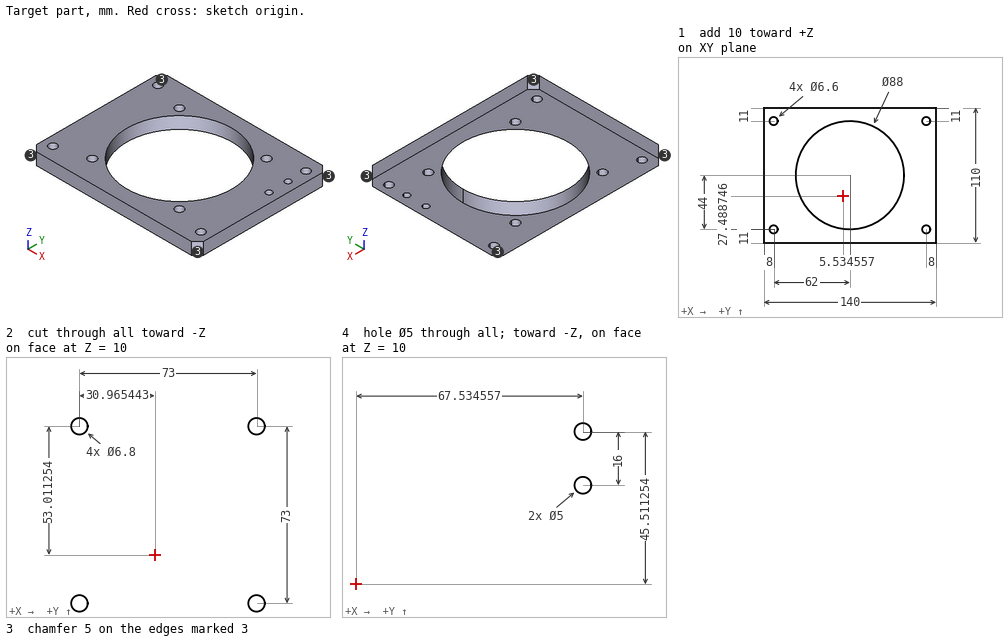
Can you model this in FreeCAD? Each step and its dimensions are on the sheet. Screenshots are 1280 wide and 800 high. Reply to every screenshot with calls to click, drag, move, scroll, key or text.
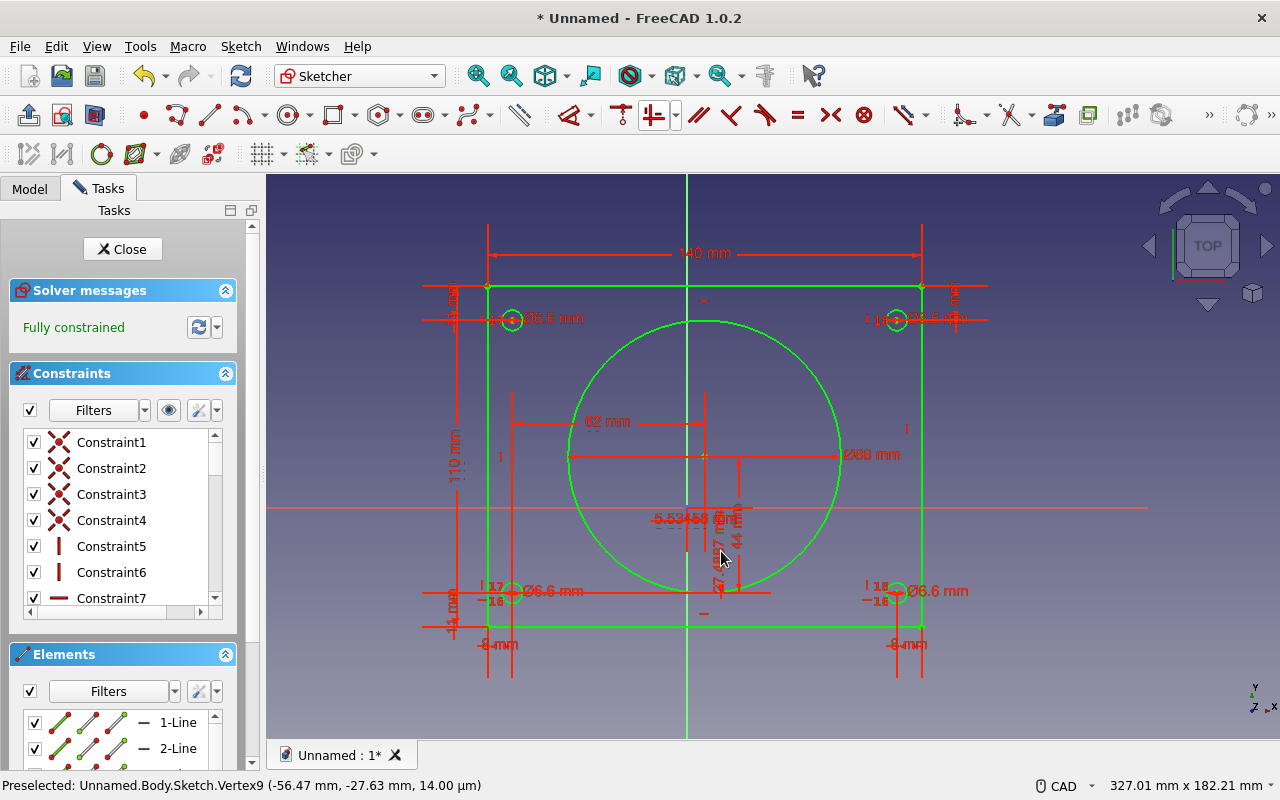
click(123, 249)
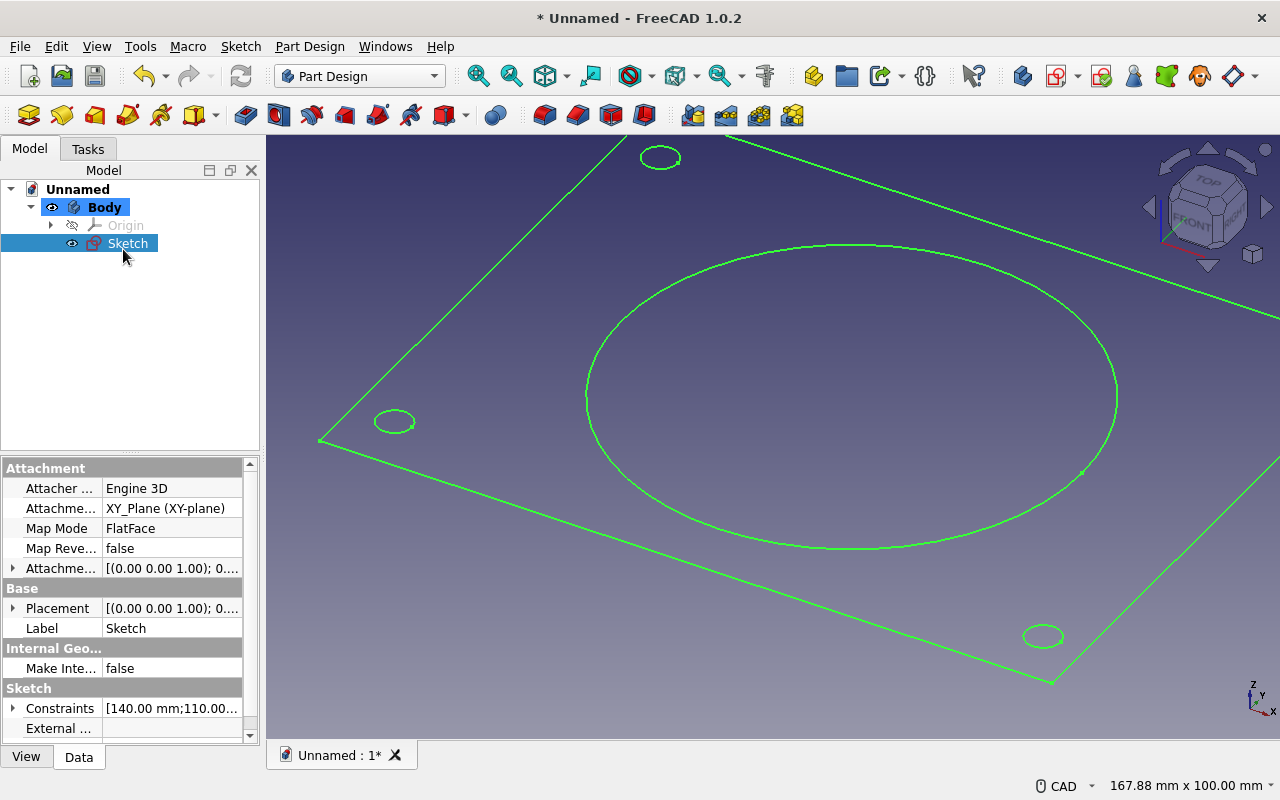
click(29, 116)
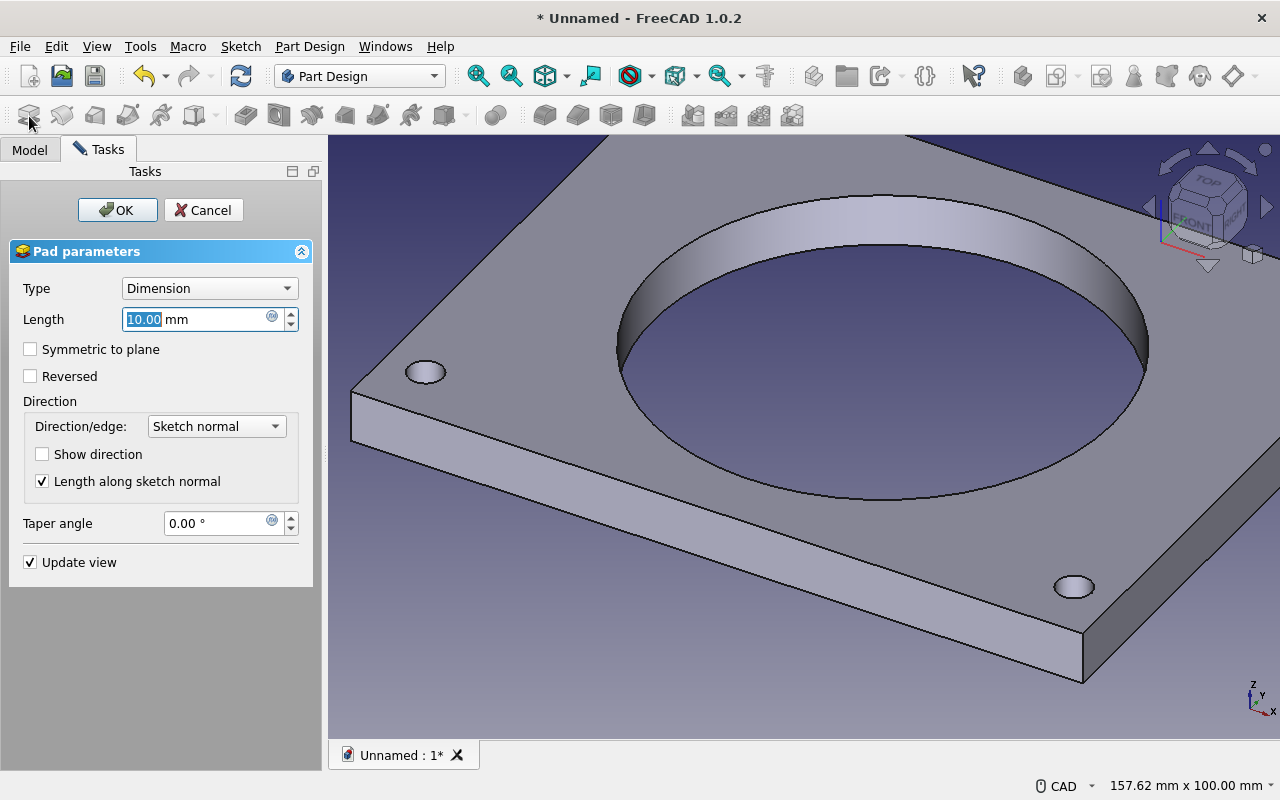
text(10)
key(Tab)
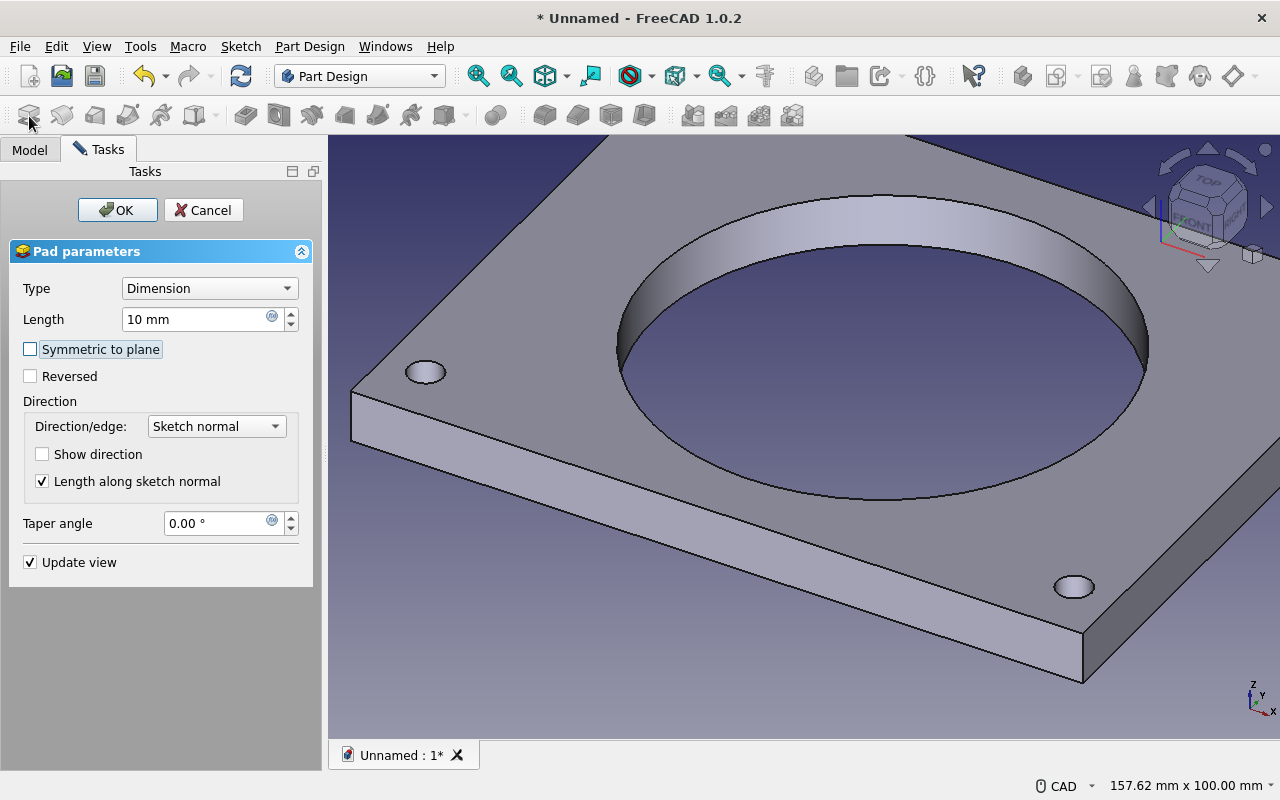
click(118, 210)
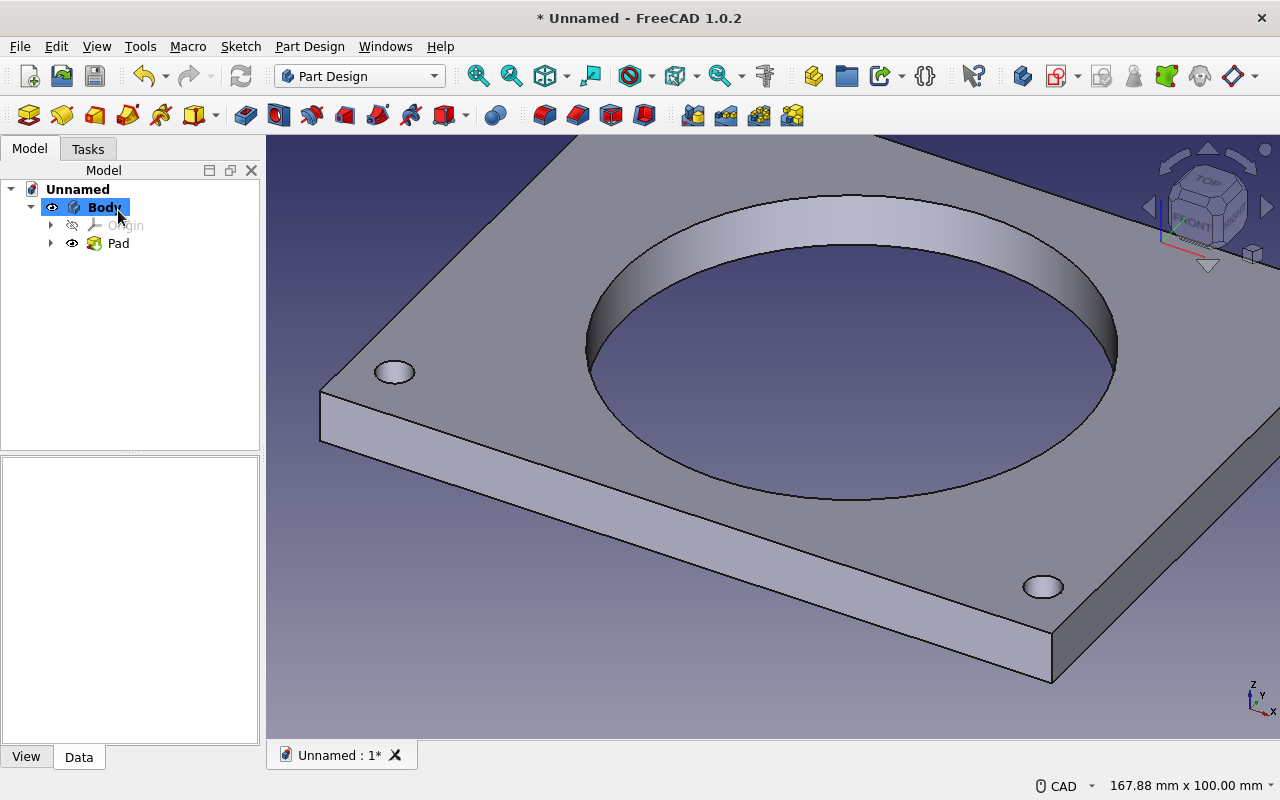
click(479, 76)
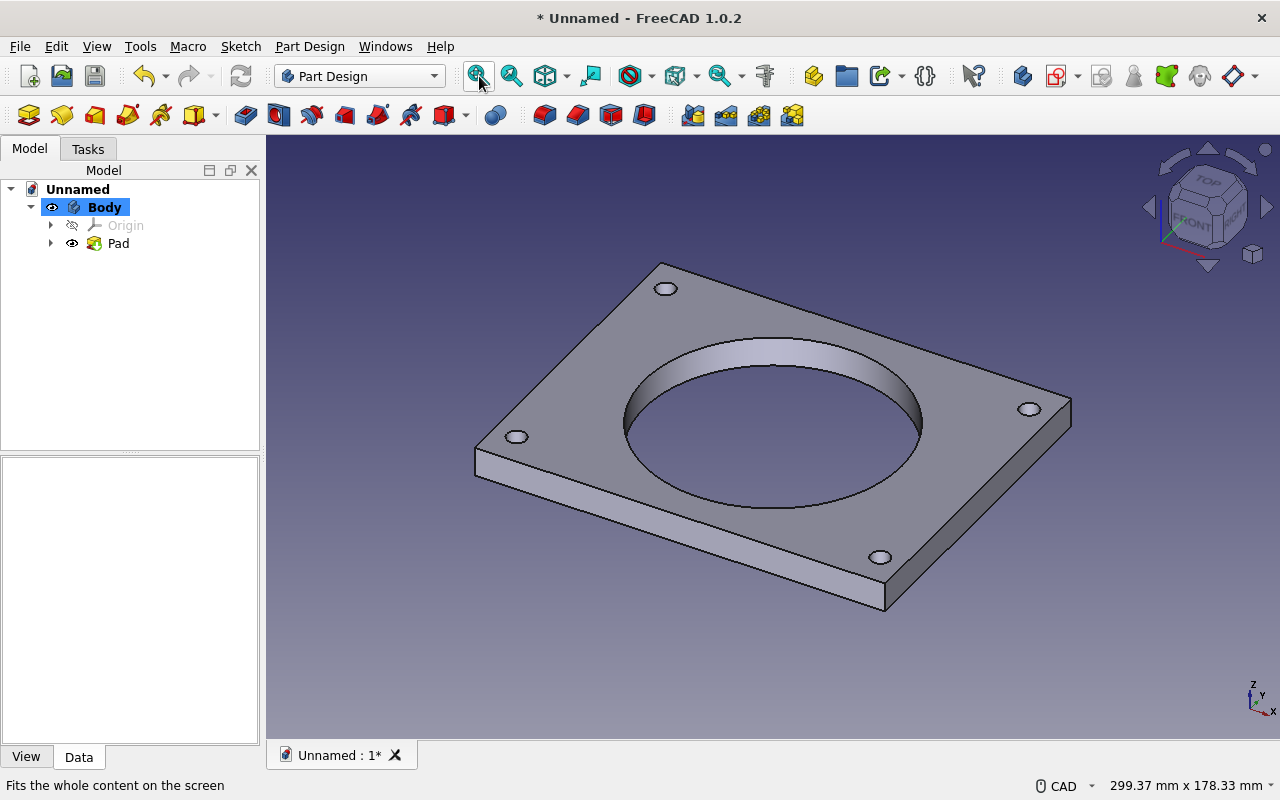
click(624, 337)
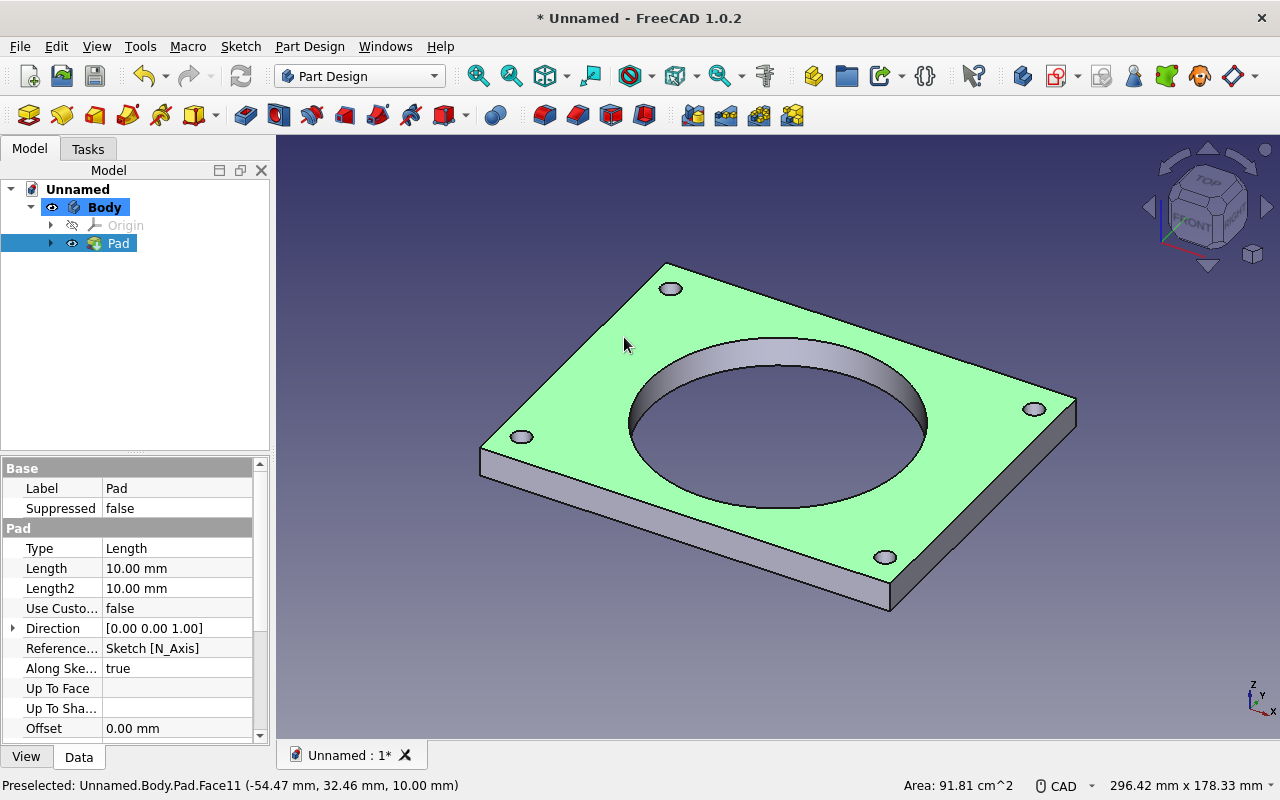
click(1056, 76)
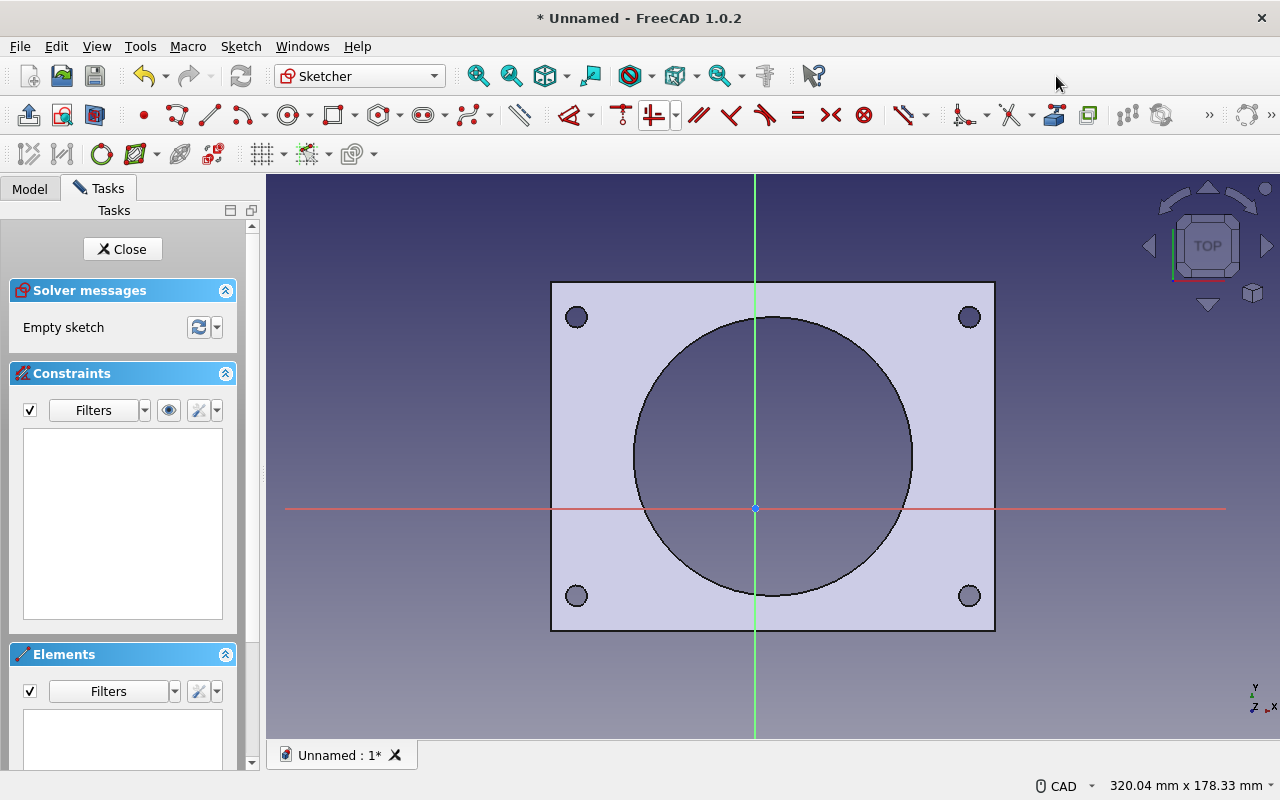
scroll(912, 456, up, 2)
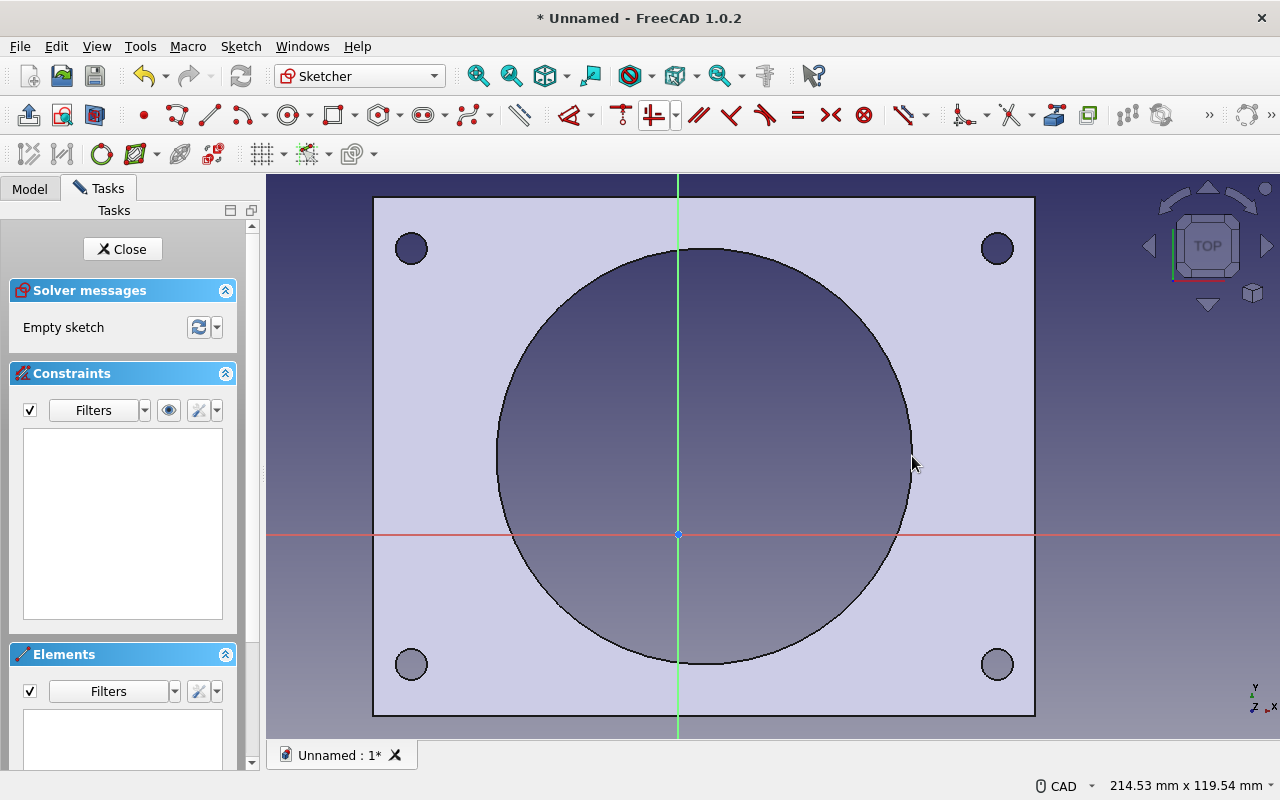
click(288, 116)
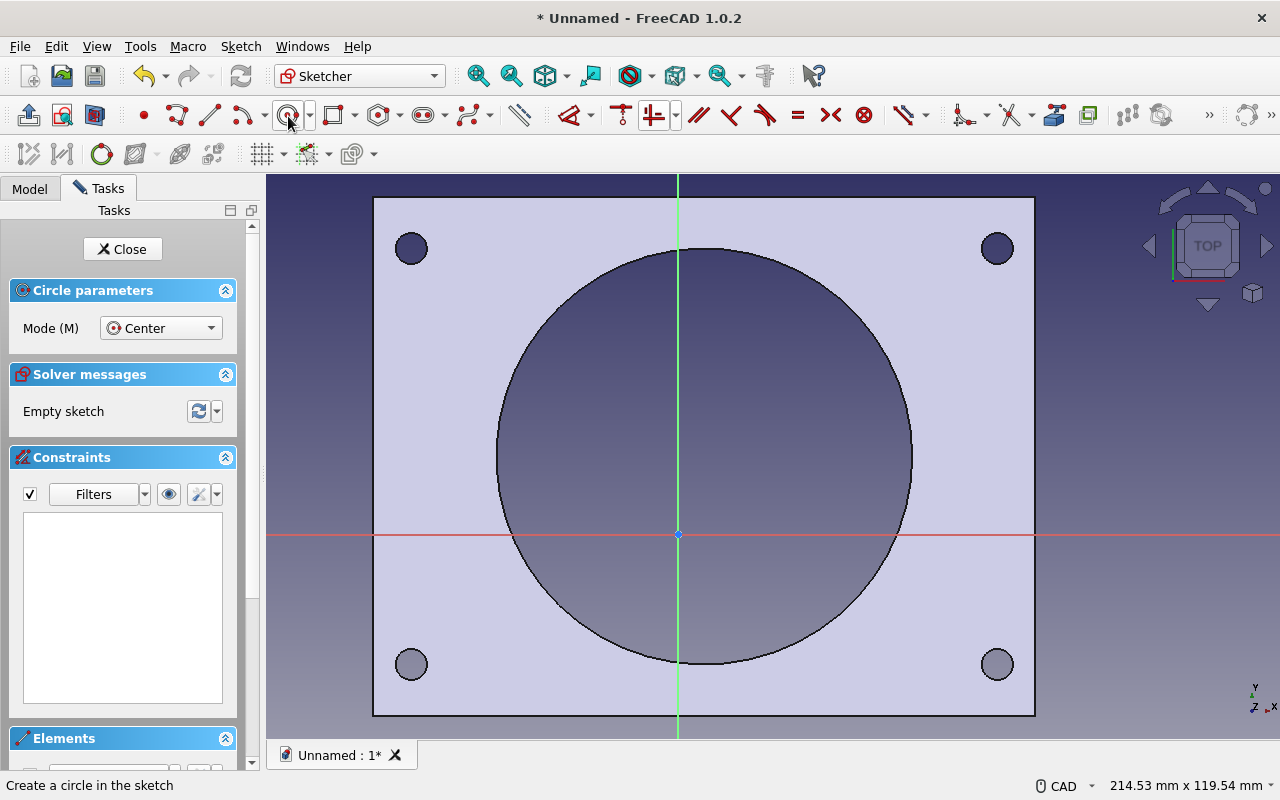
scroll(532, 284, up, 2)